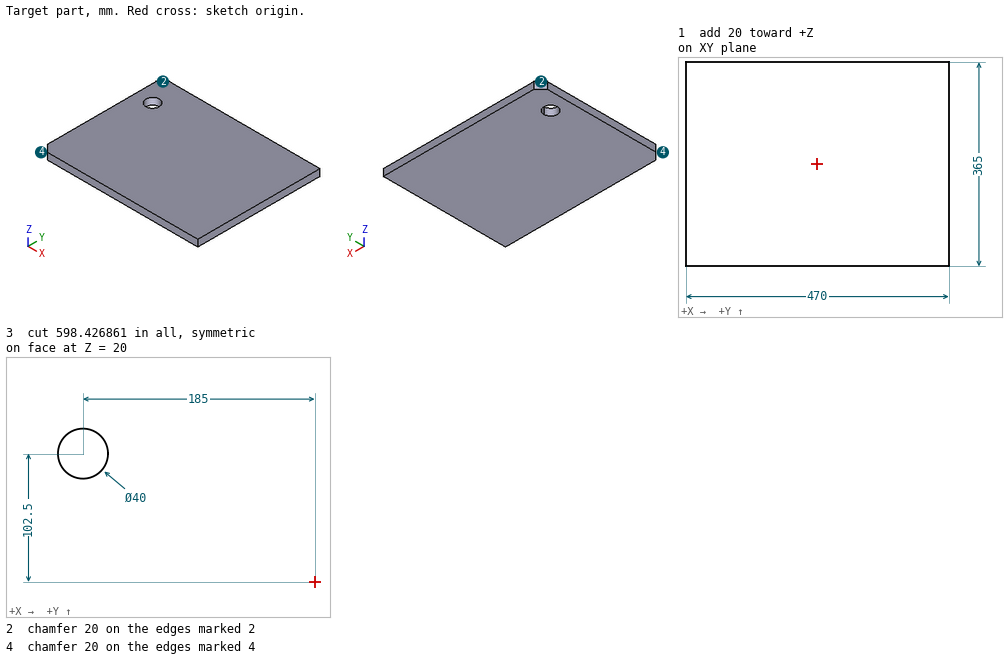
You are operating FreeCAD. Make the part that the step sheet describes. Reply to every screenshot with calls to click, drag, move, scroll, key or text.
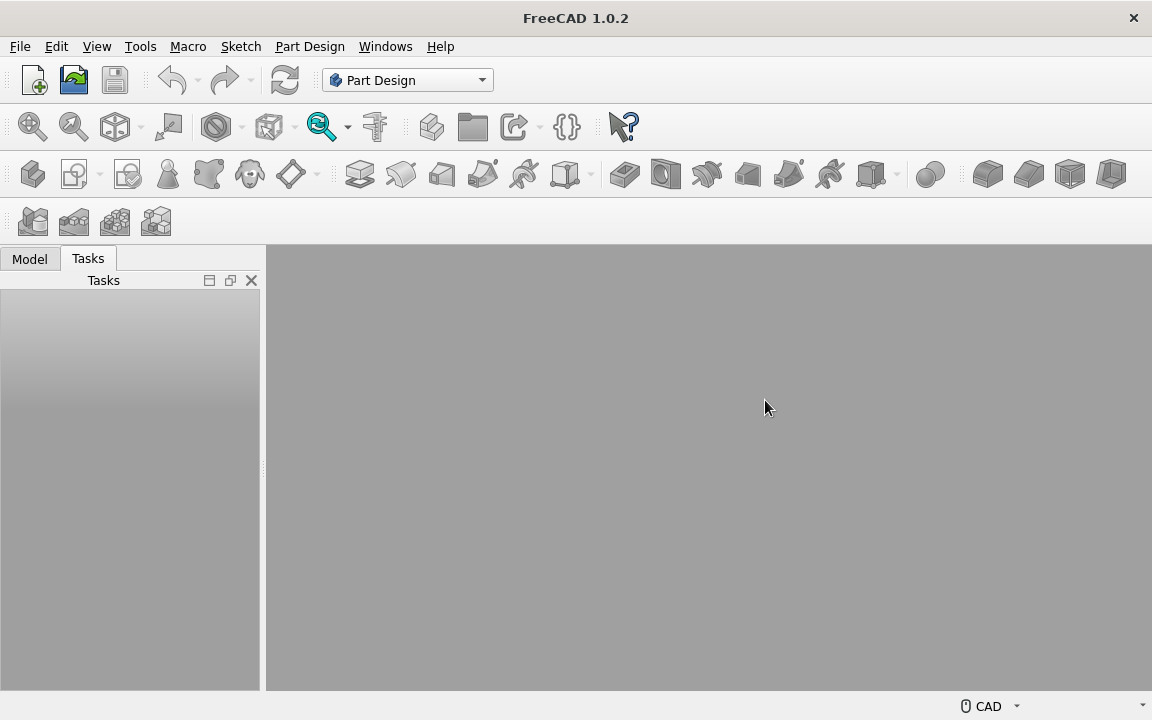
click(33, 80)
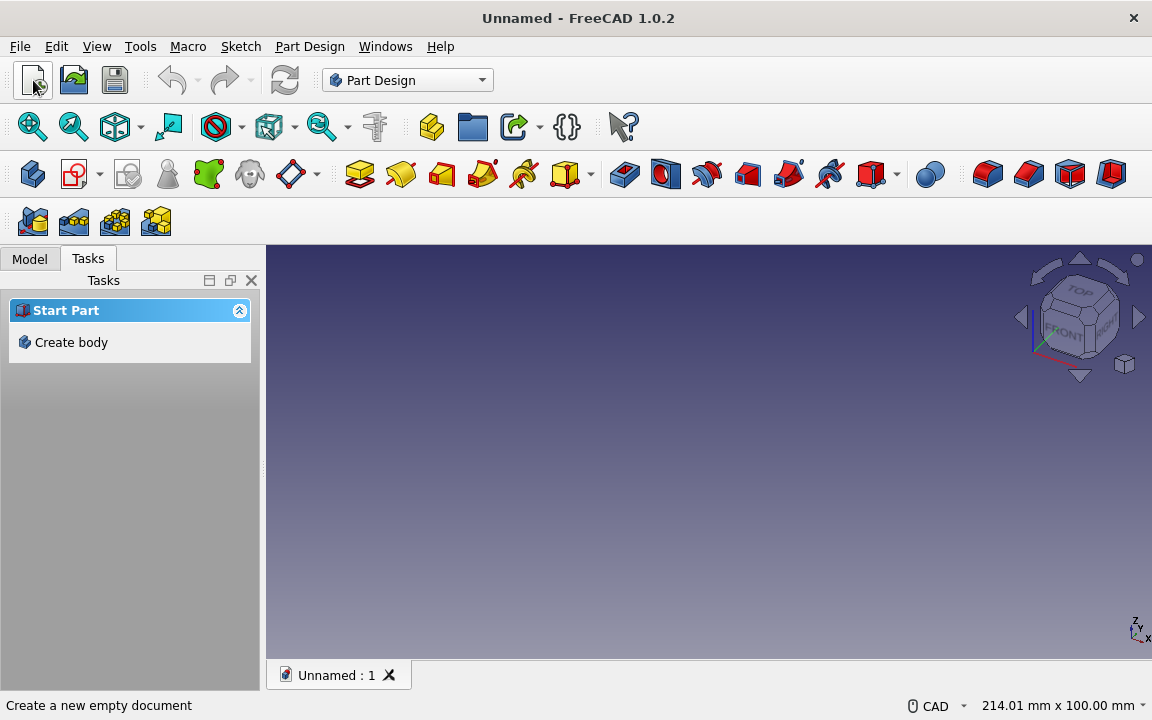
click(74, 174)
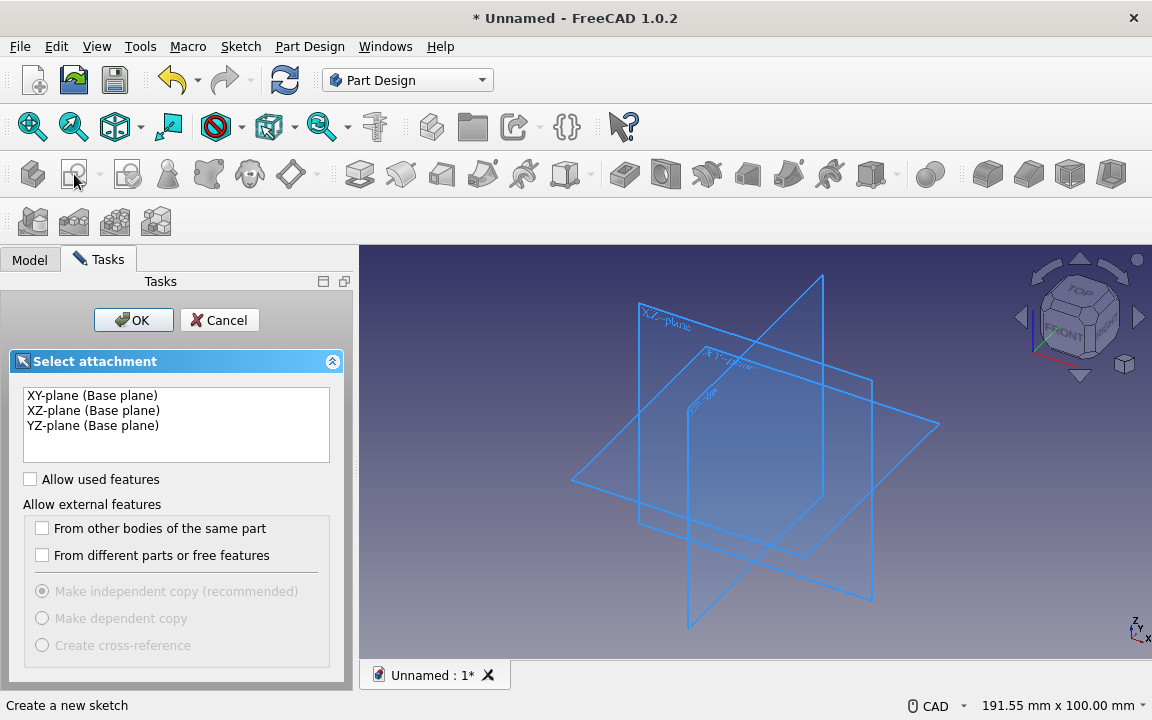
click(84, 396)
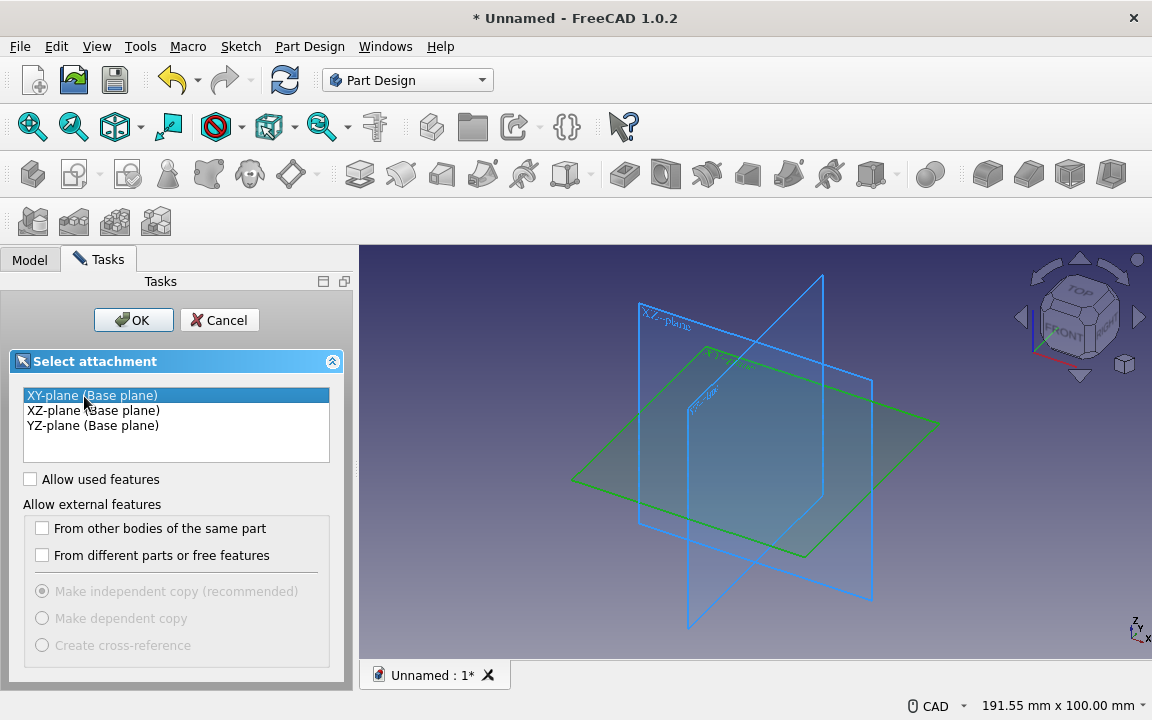
click(134, 320)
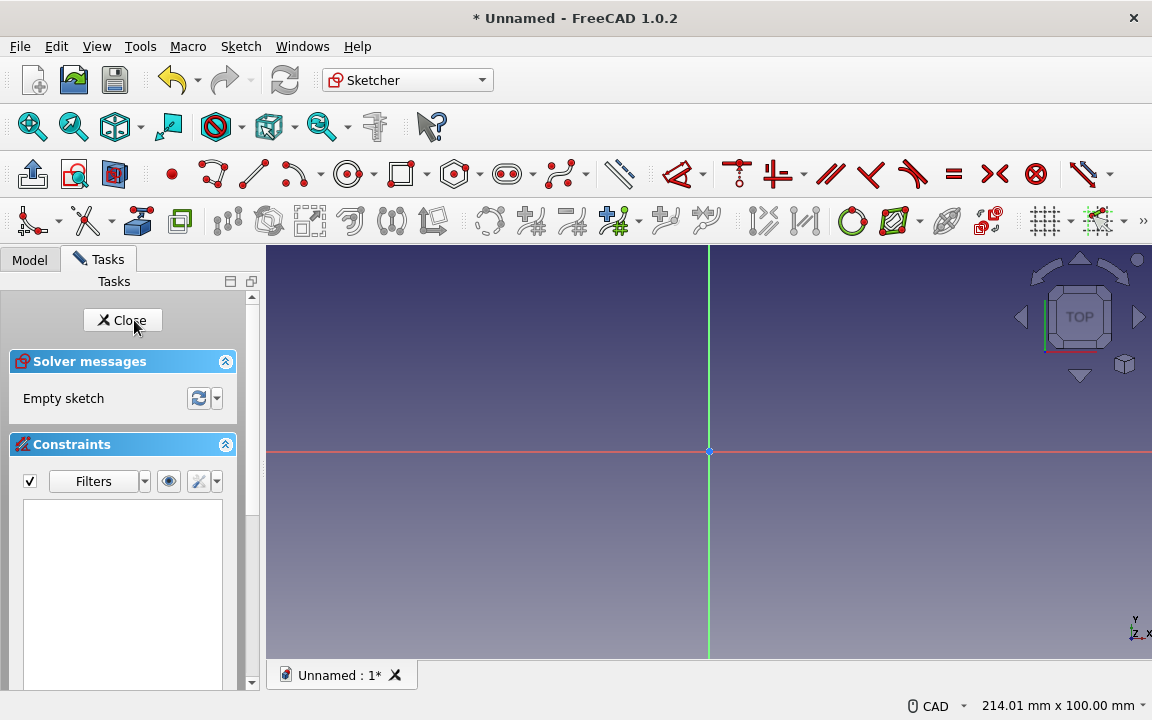
scroll(627, 452, down, 9)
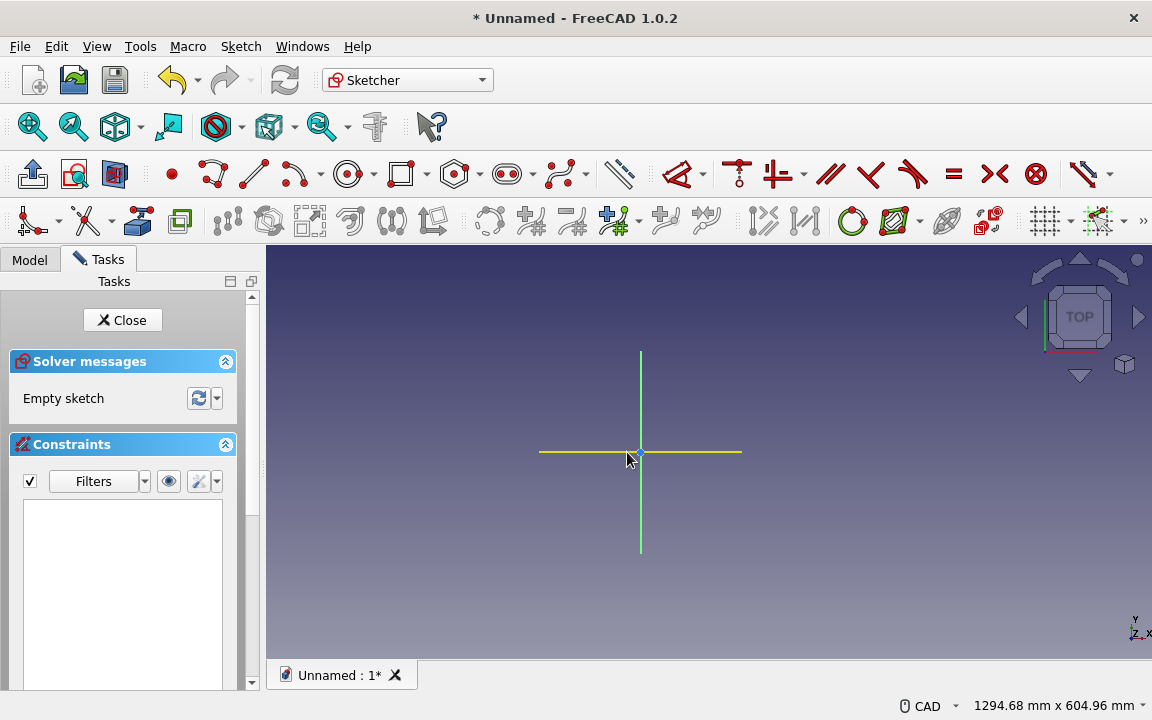
click(426, 174)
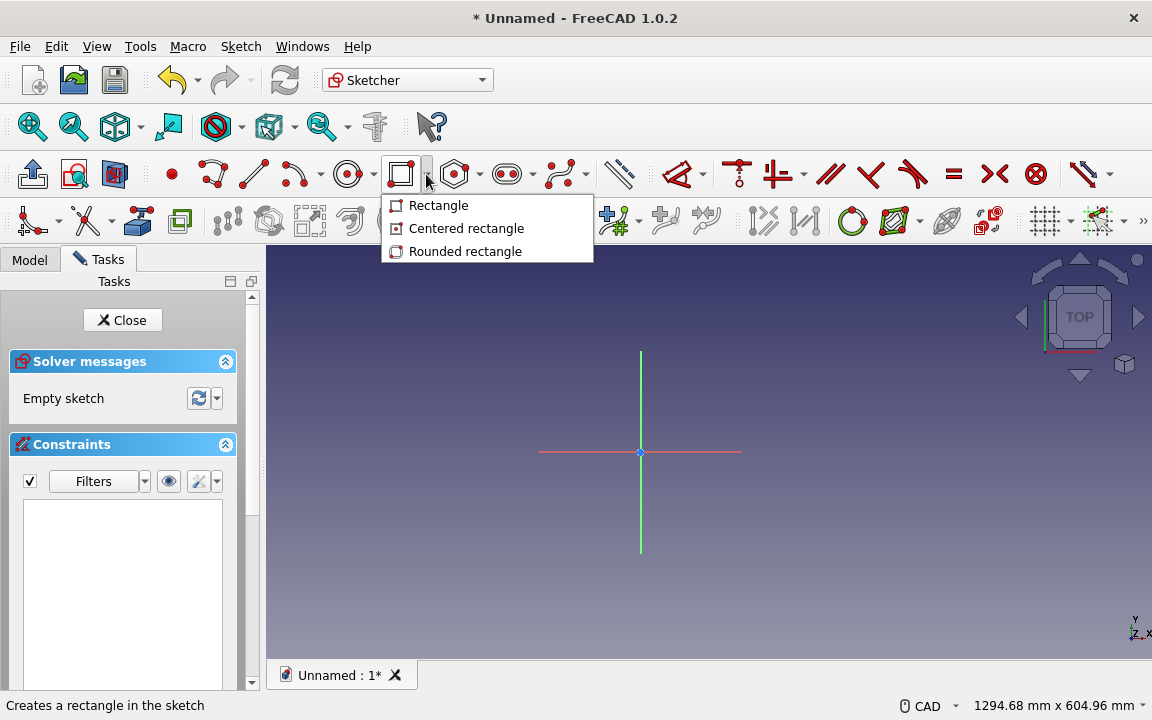
click(488, 228)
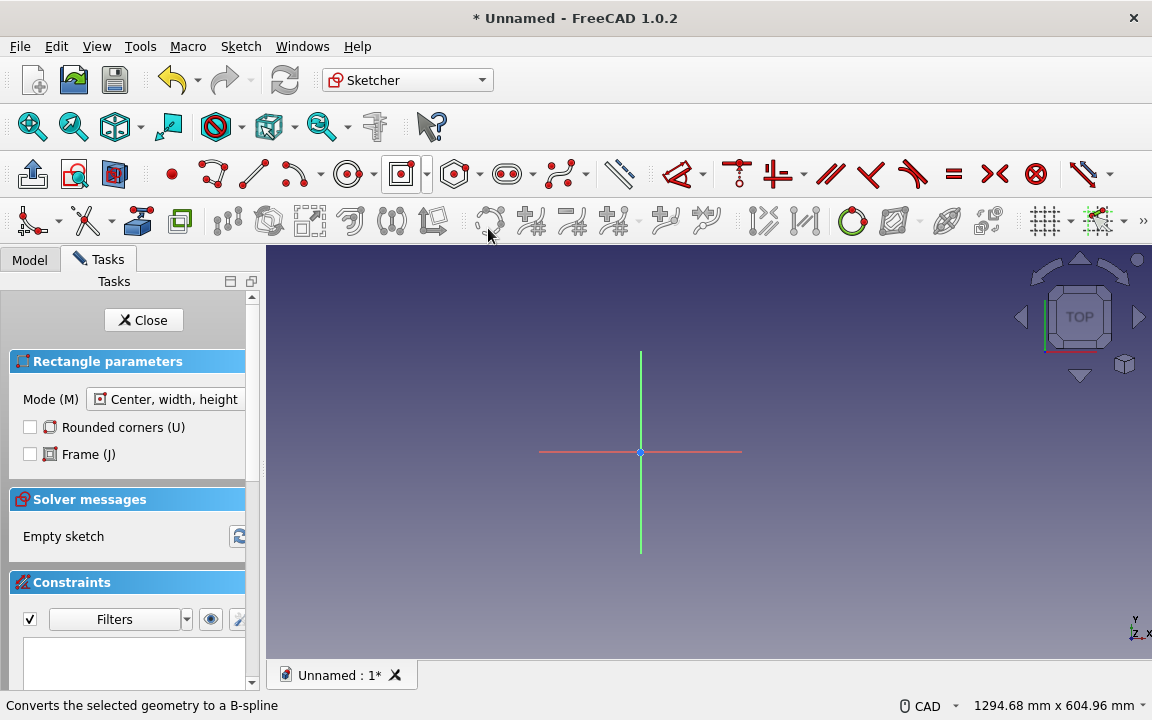
click(641, 452)
click(802, 328)
key(Escape)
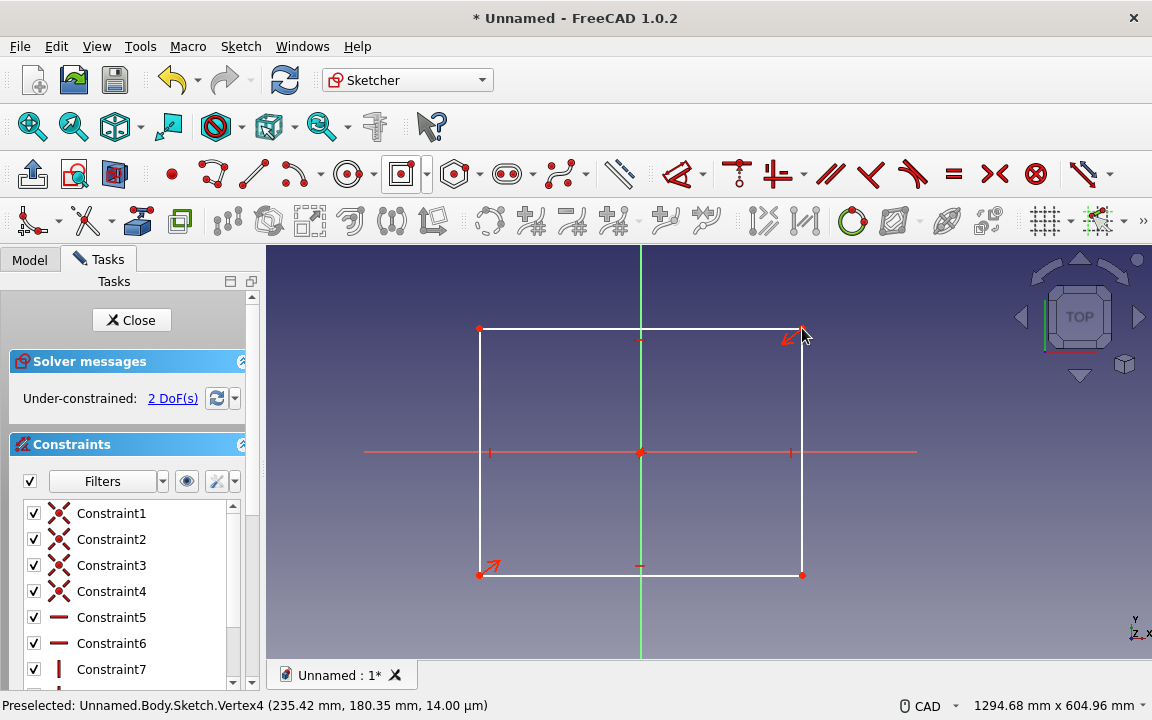
click(676, 174)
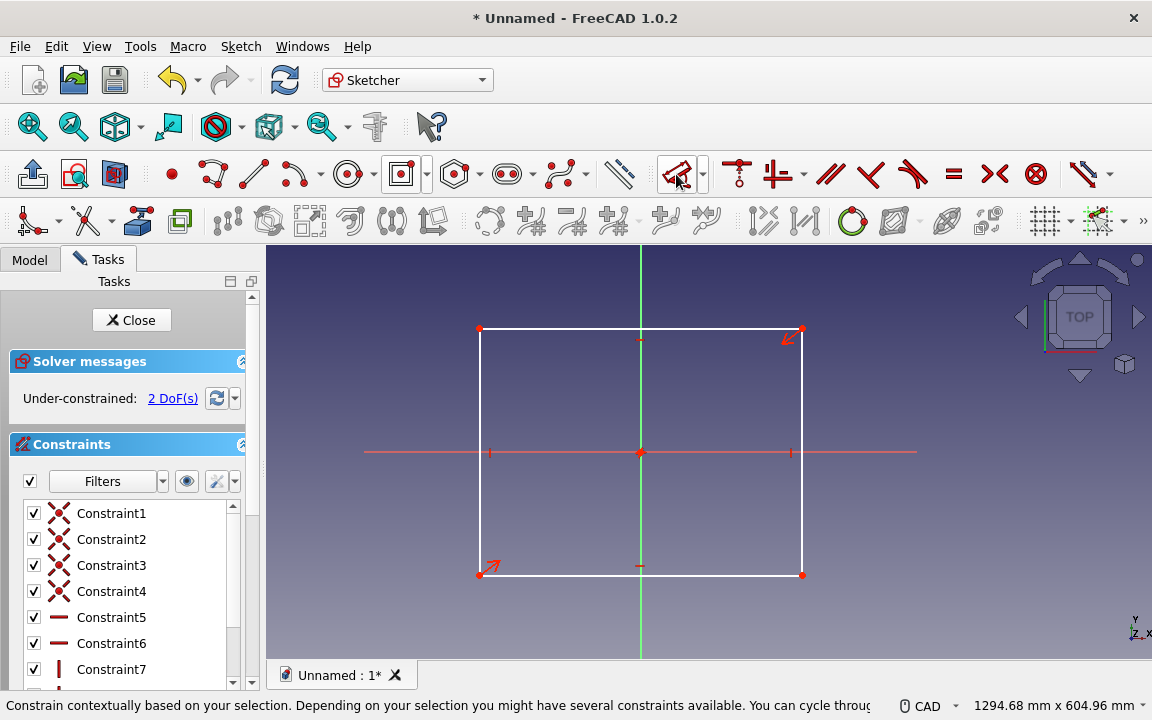
click(576, 576)
click(567, 610)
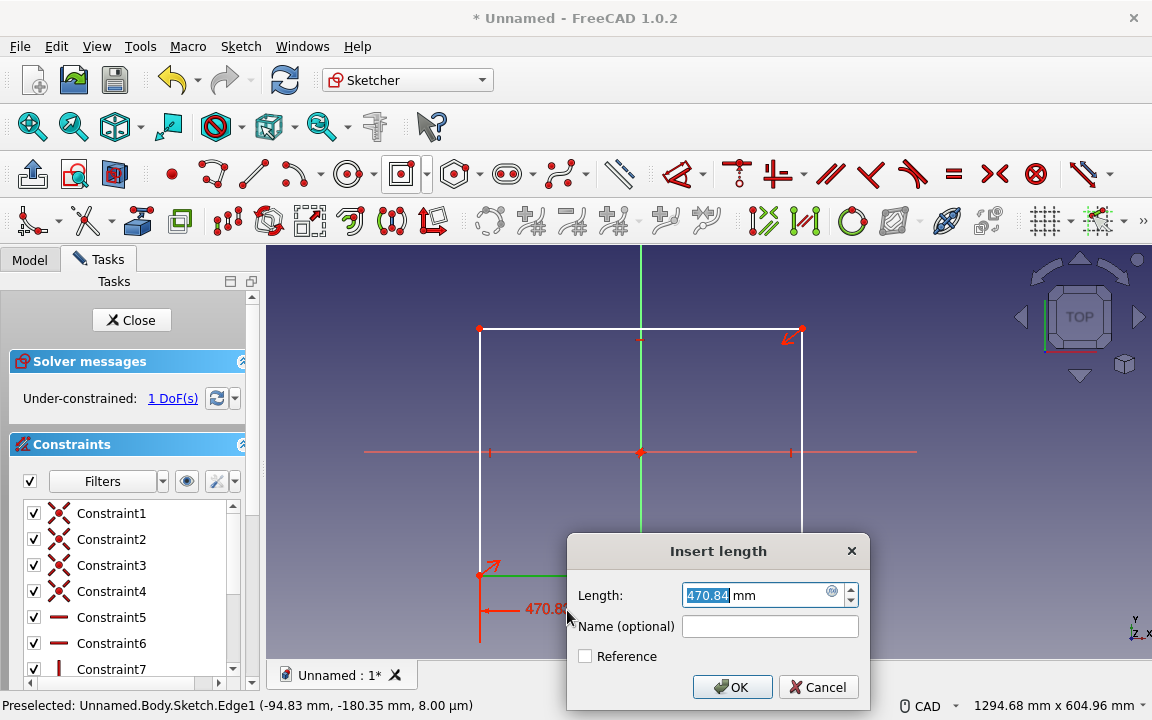
text(470)
key(Return)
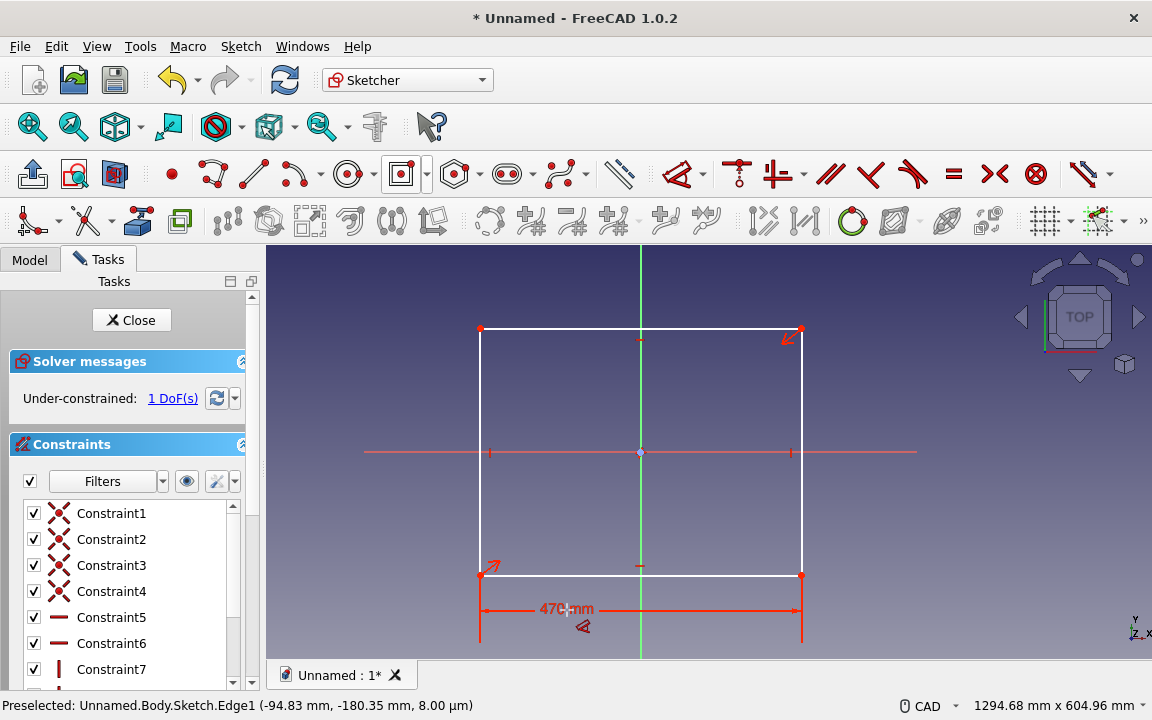
click(802, 502)
click(836, 396)